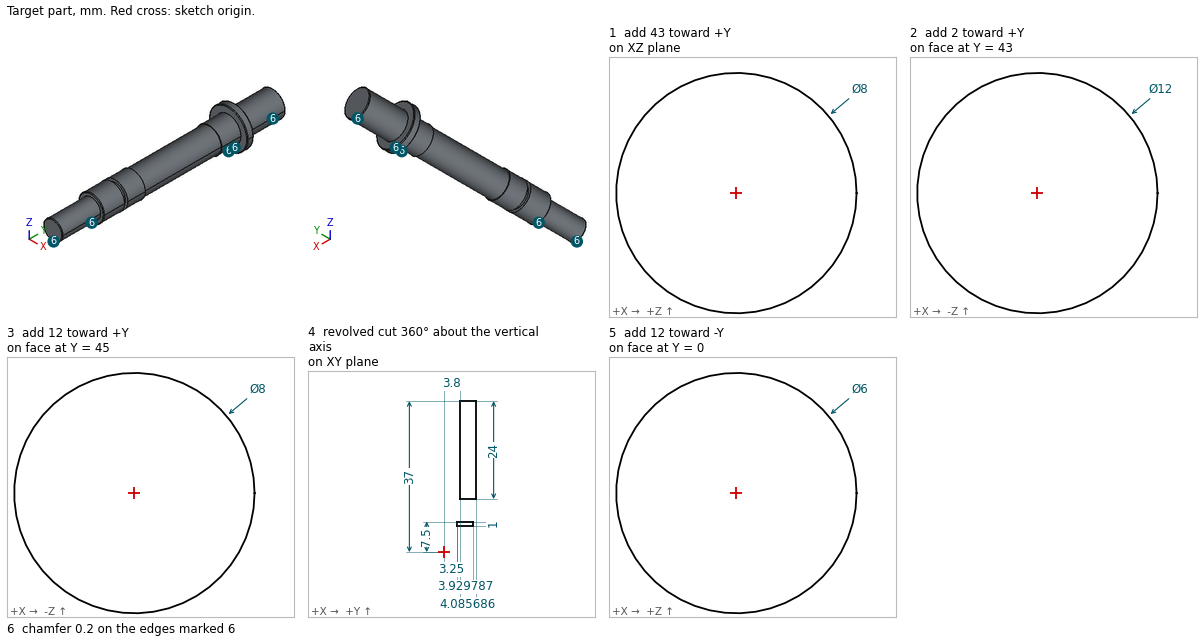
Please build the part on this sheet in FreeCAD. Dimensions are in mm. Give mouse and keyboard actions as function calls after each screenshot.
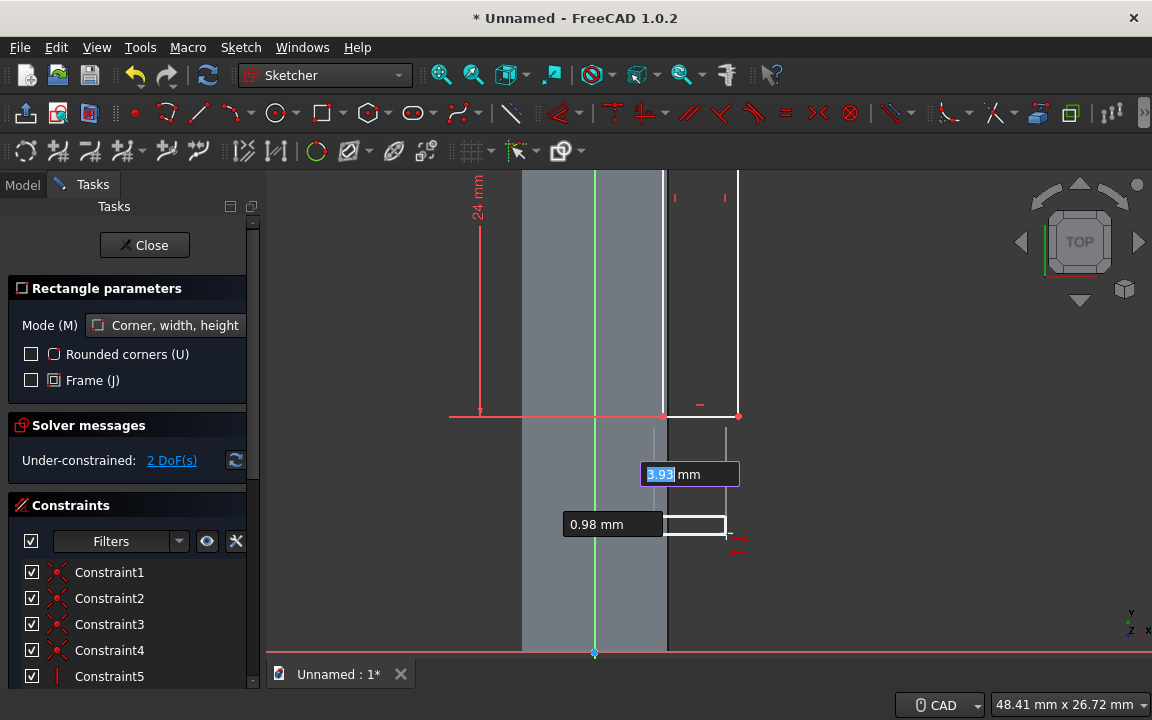
text(3.929787)
key(Tab)
text(1)
key(Return)
key(Escape)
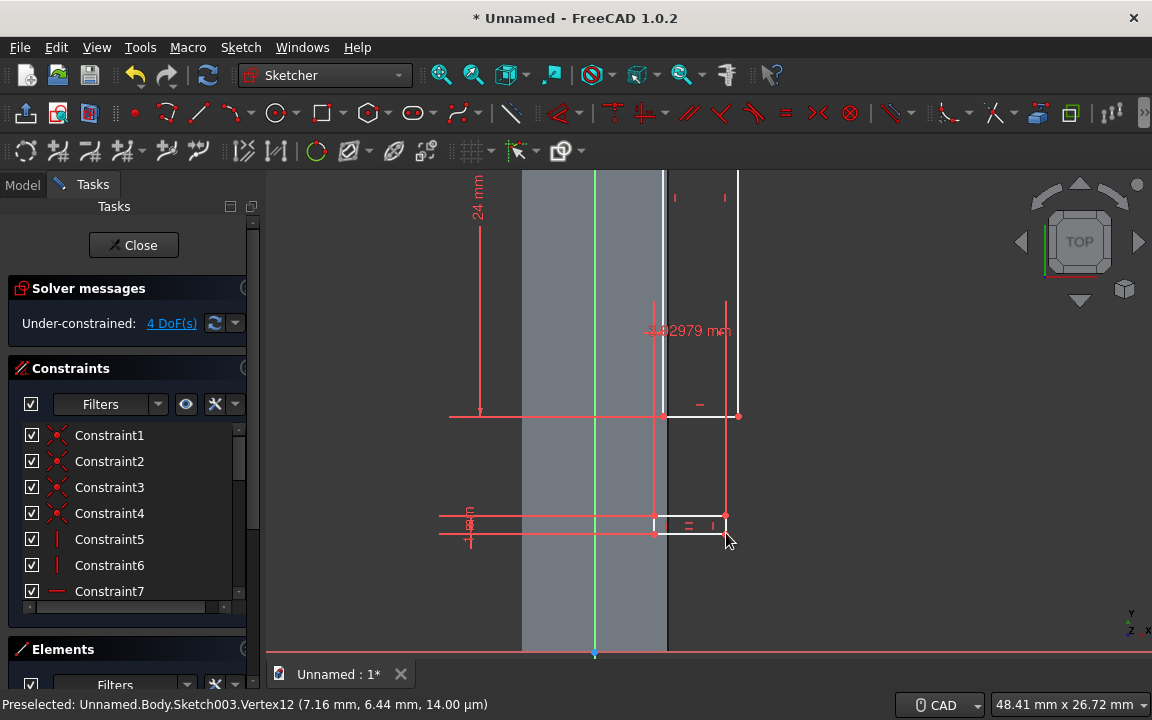
scroll(619, 497, down, 4)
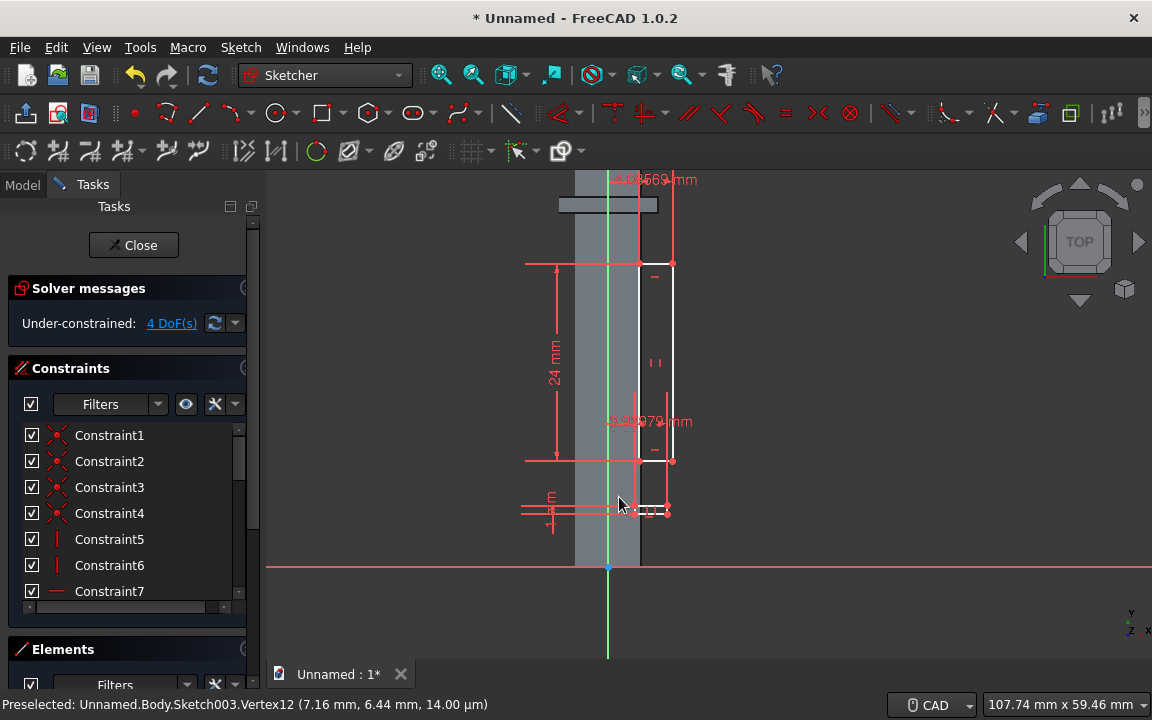
click(639, 264)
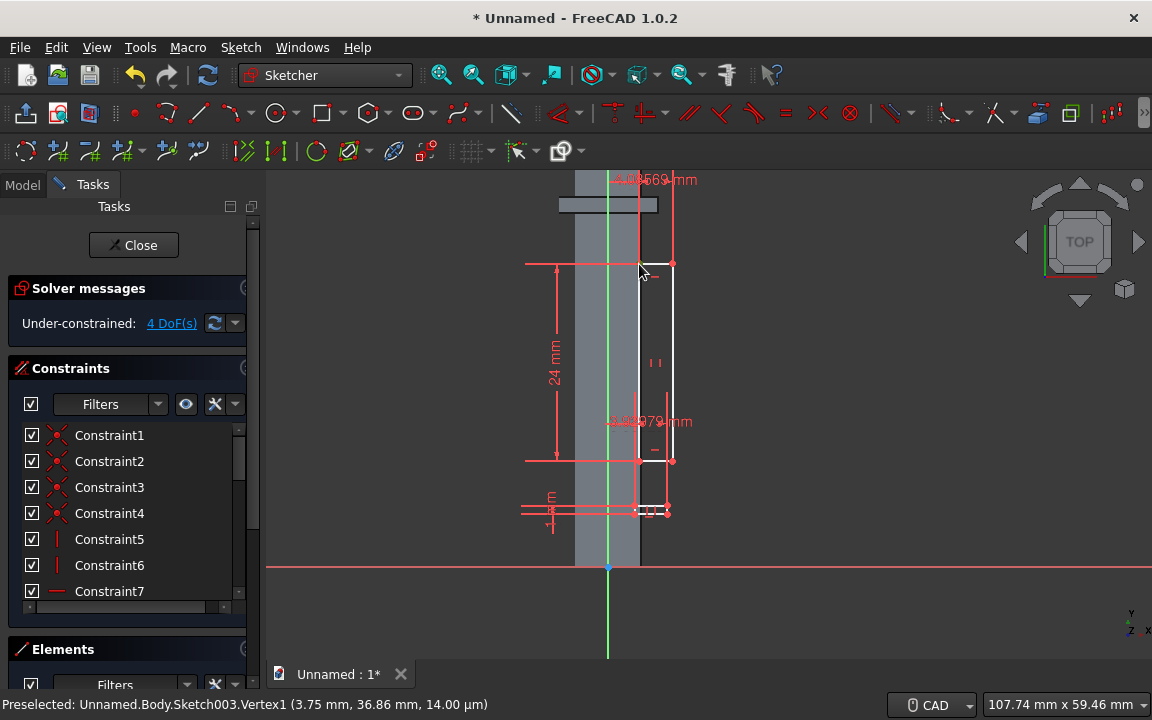
key(i)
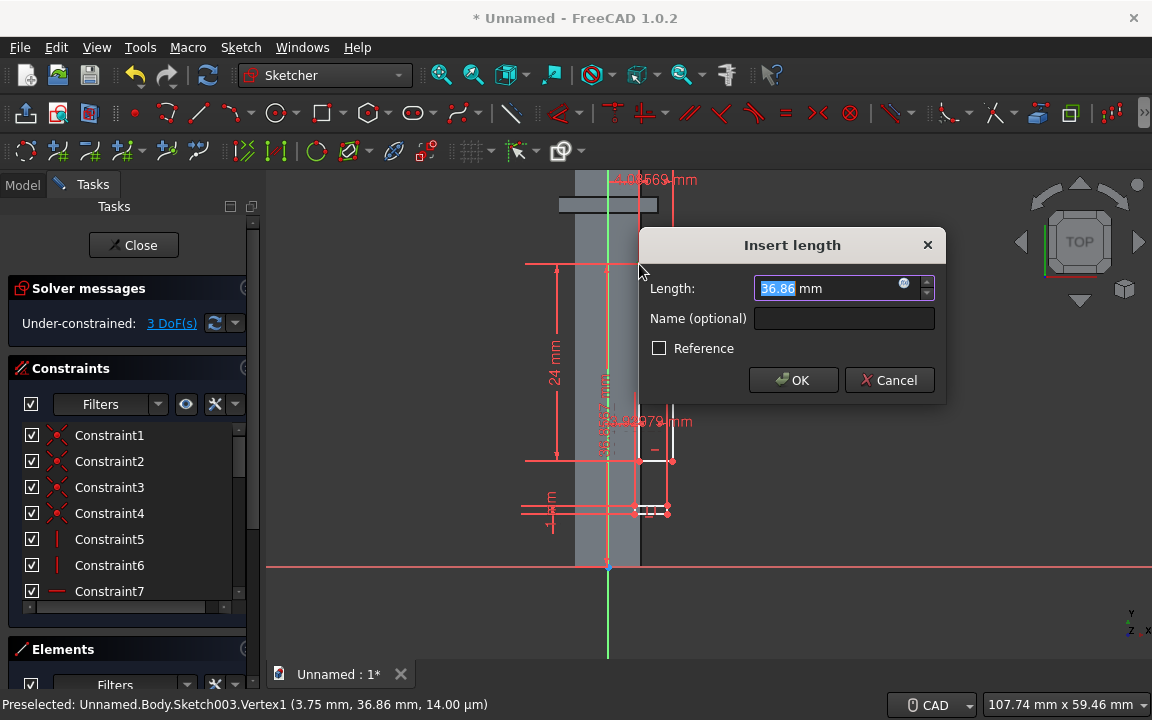
text(37)
key(Return)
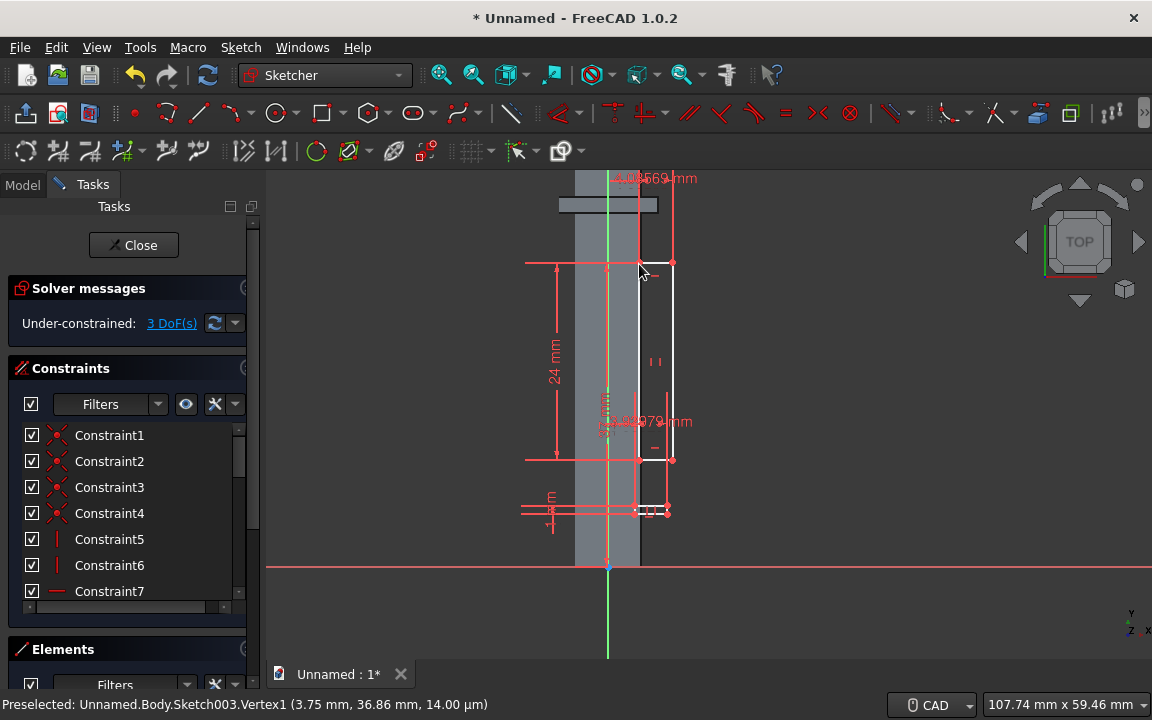
scroll(639, 263, up, 2)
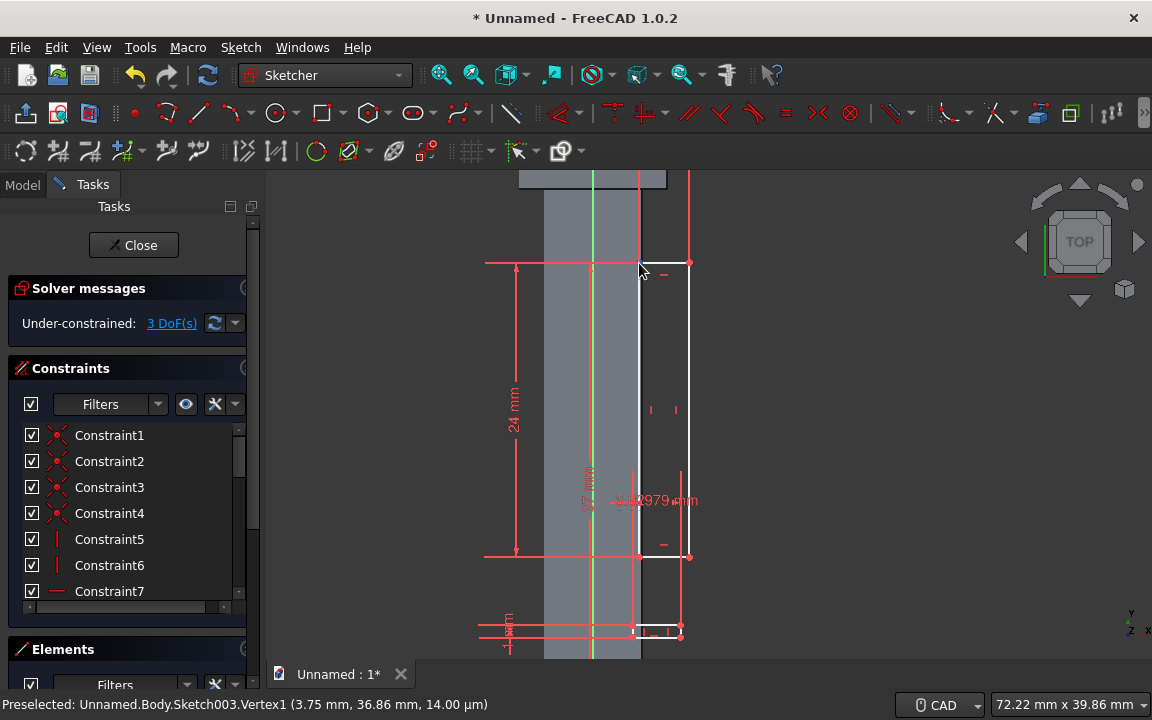
click(639, 263)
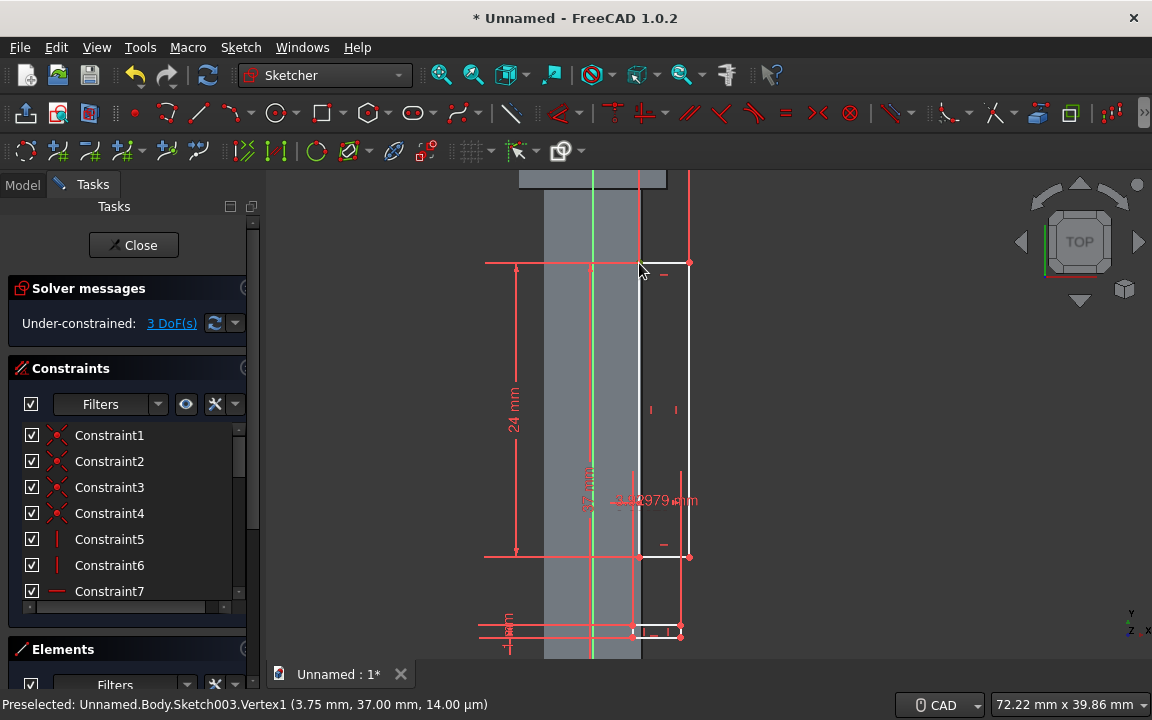
key(l)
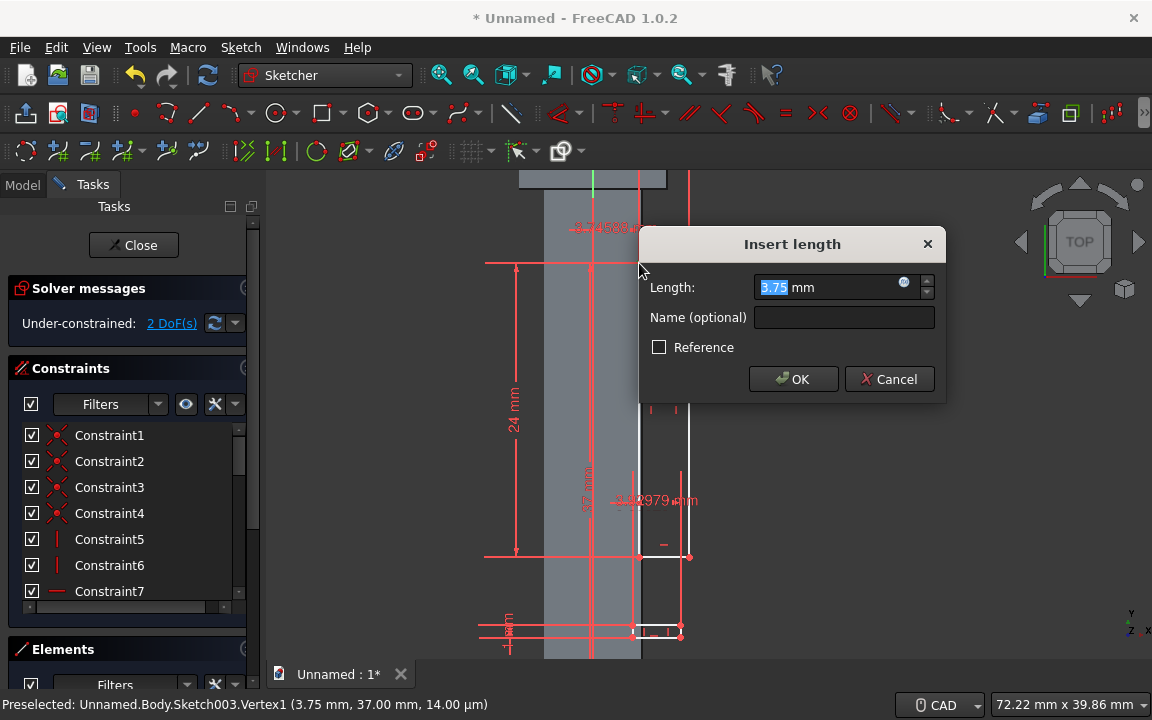
text(3.8)
key(Return)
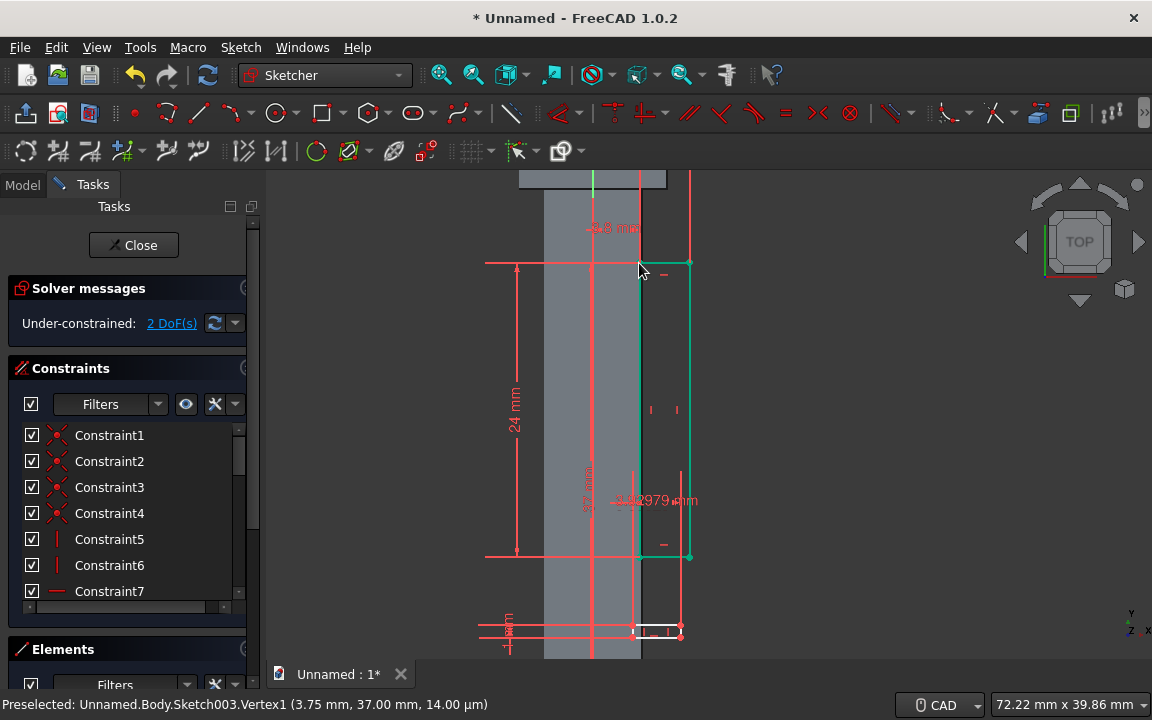
click(633, 625)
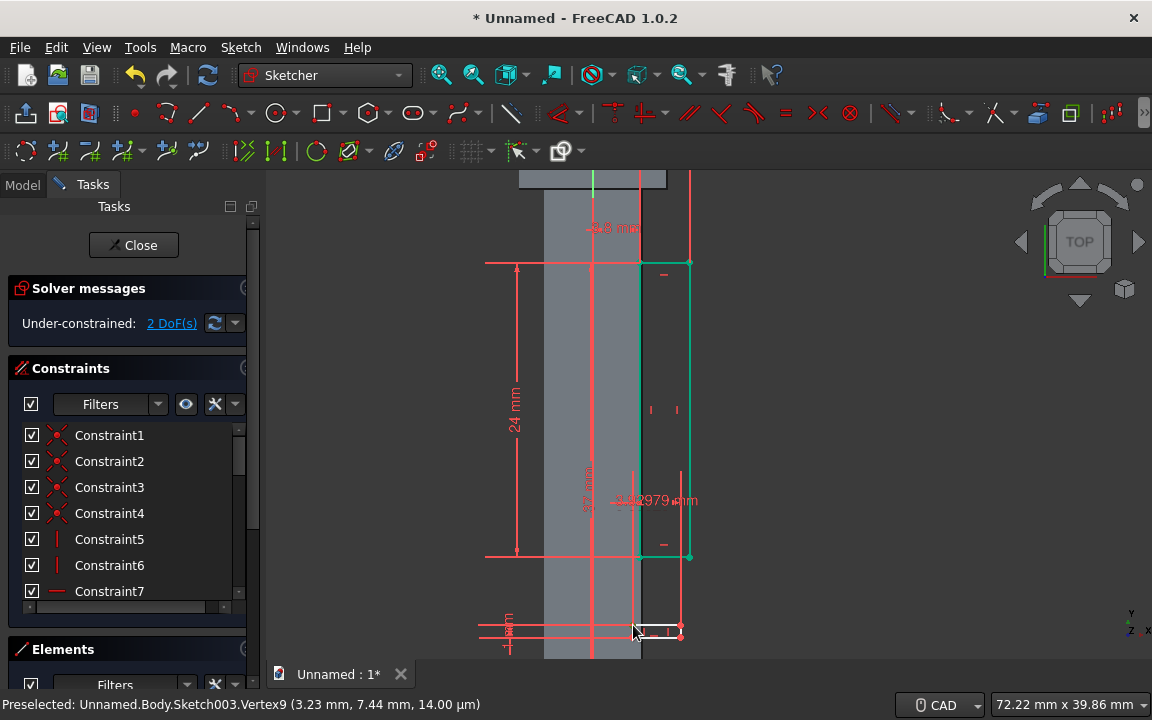
key(i)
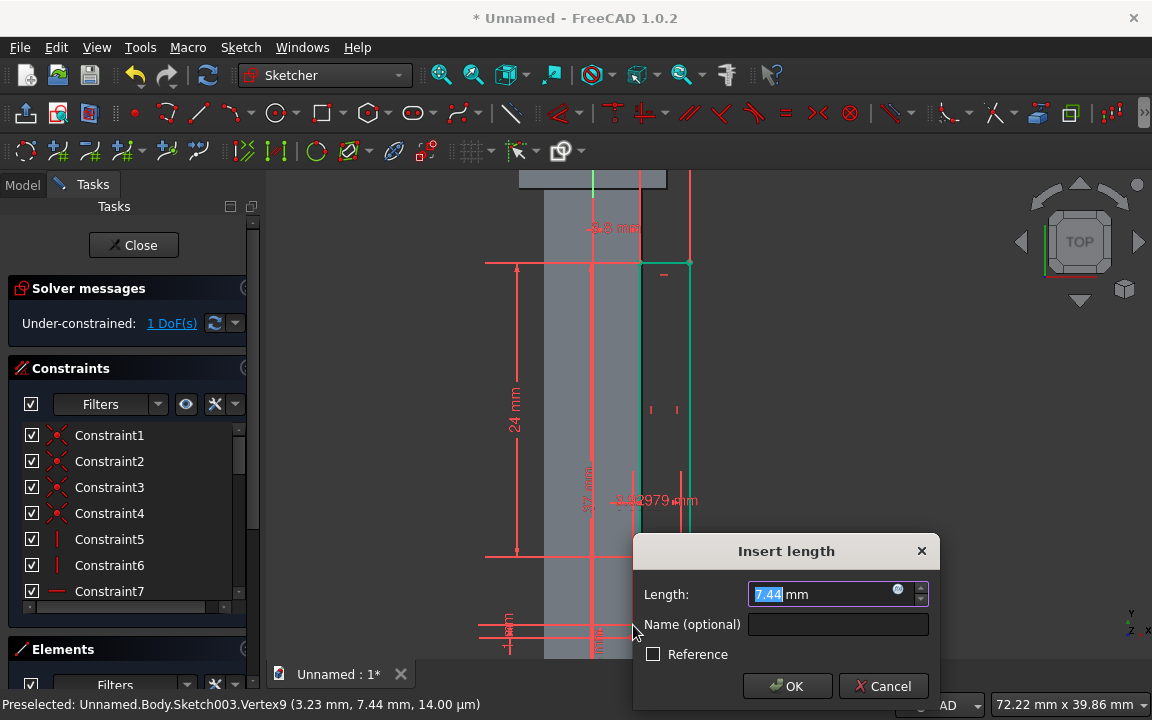
text(7.5)
key(Return)